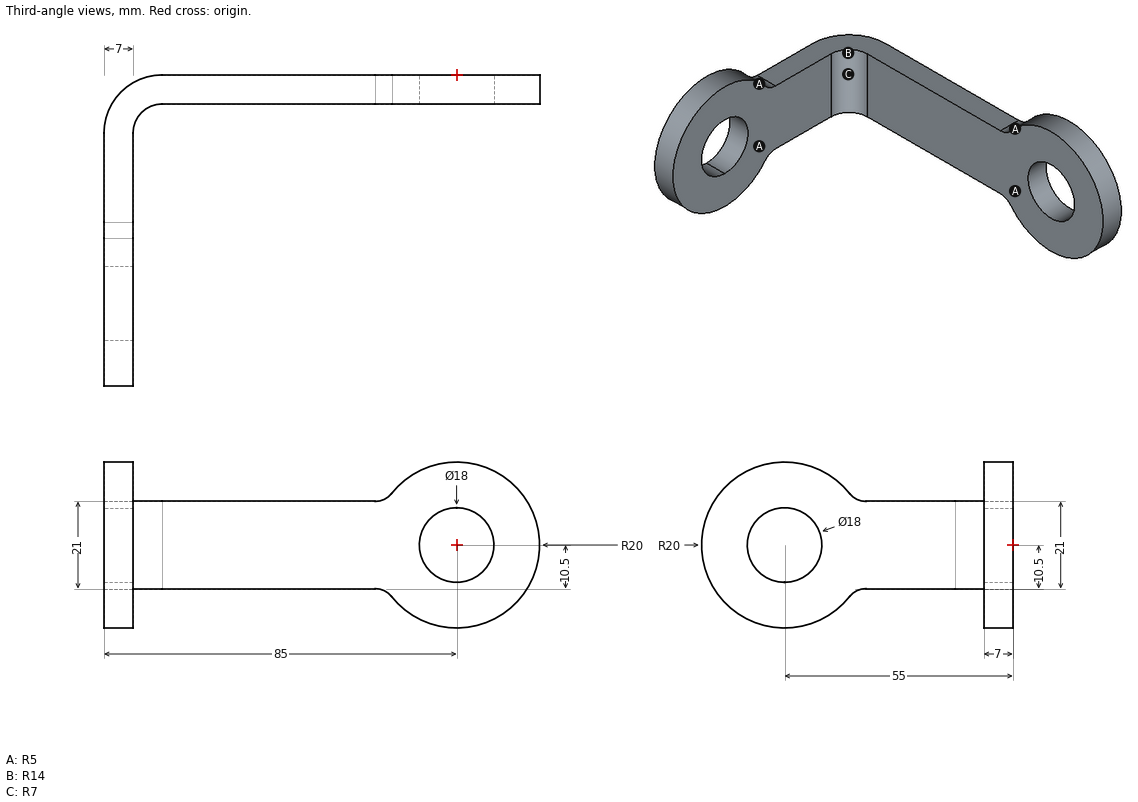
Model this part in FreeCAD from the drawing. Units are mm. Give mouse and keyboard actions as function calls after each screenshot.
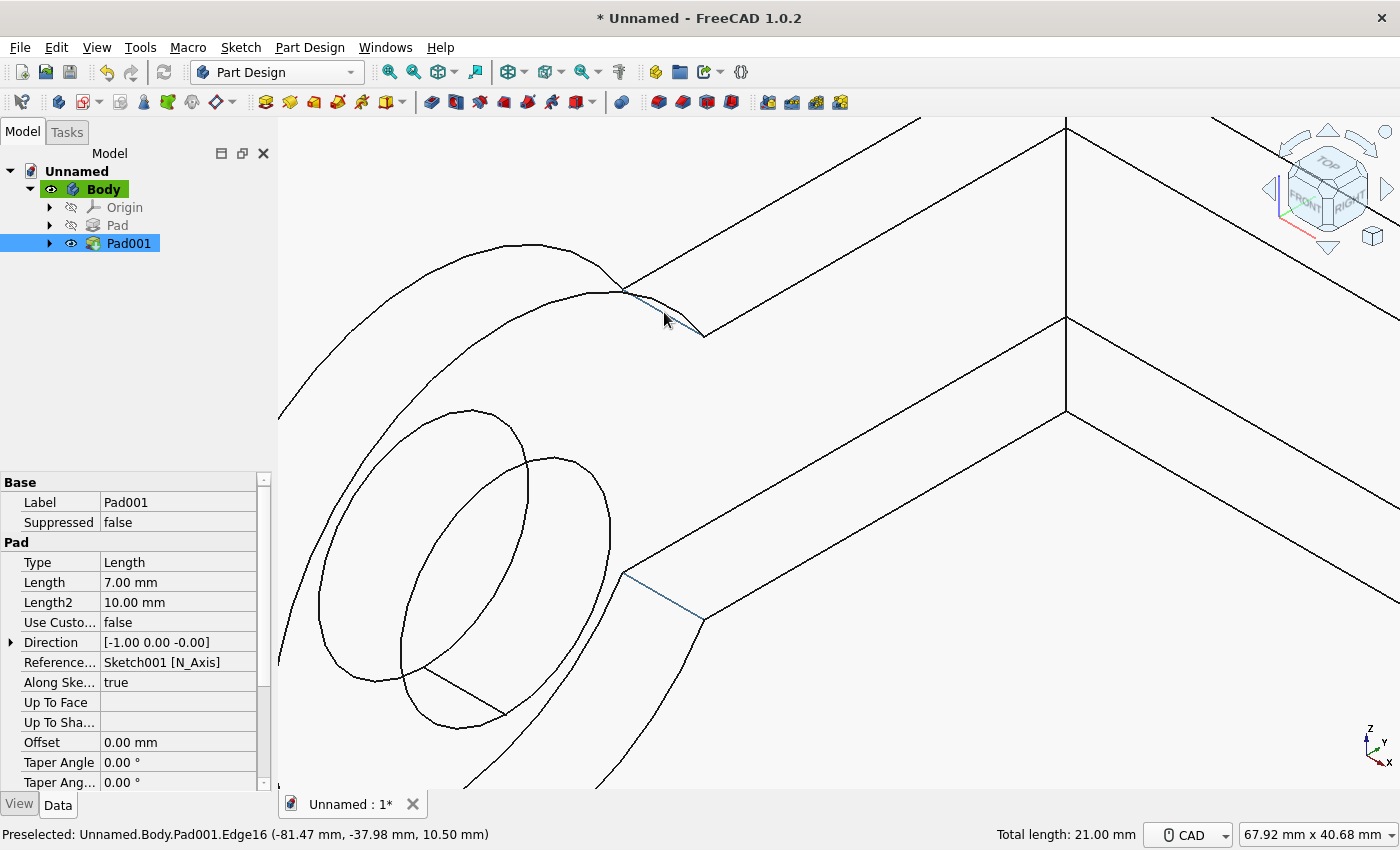
click(390, 72)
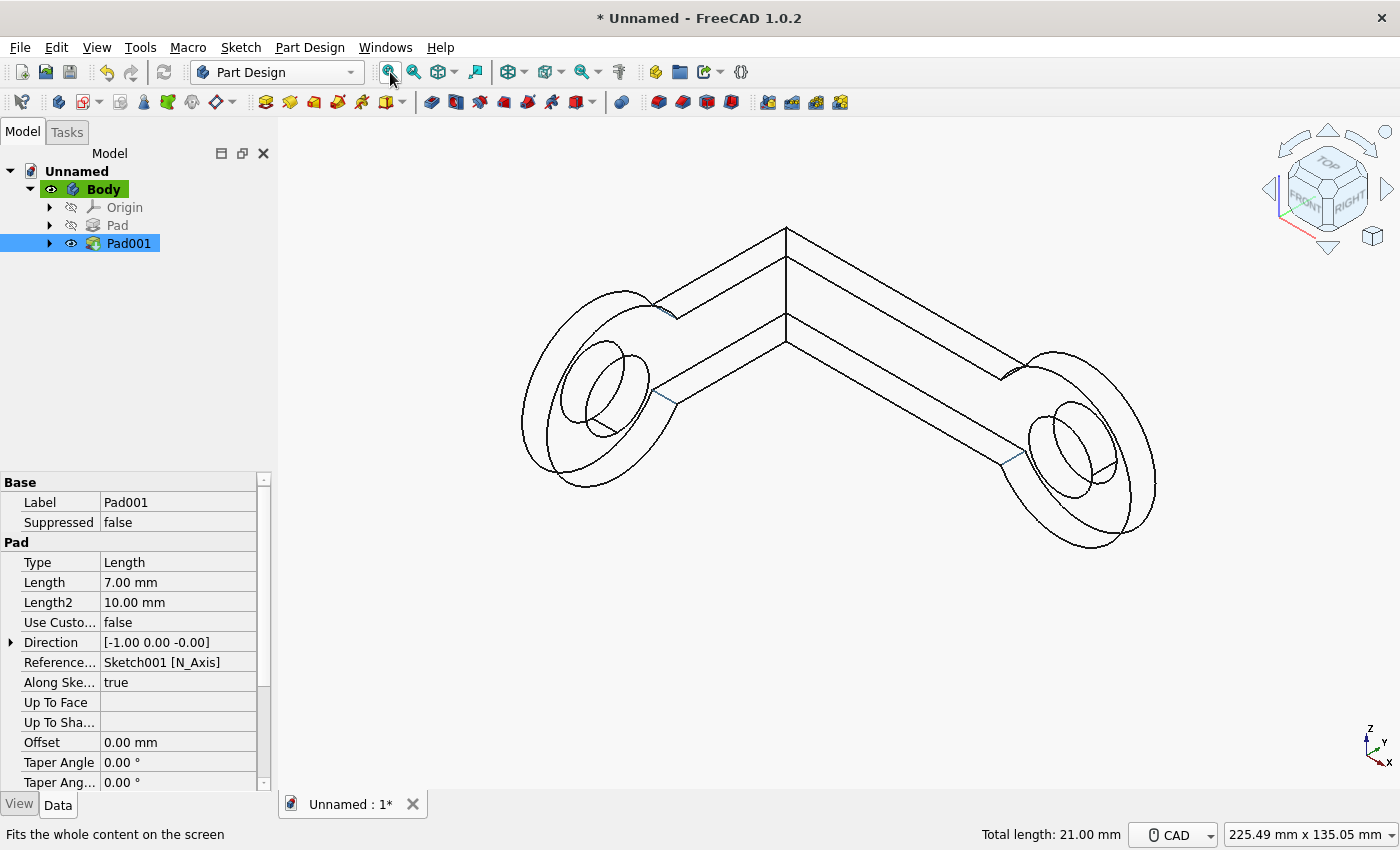
key(2)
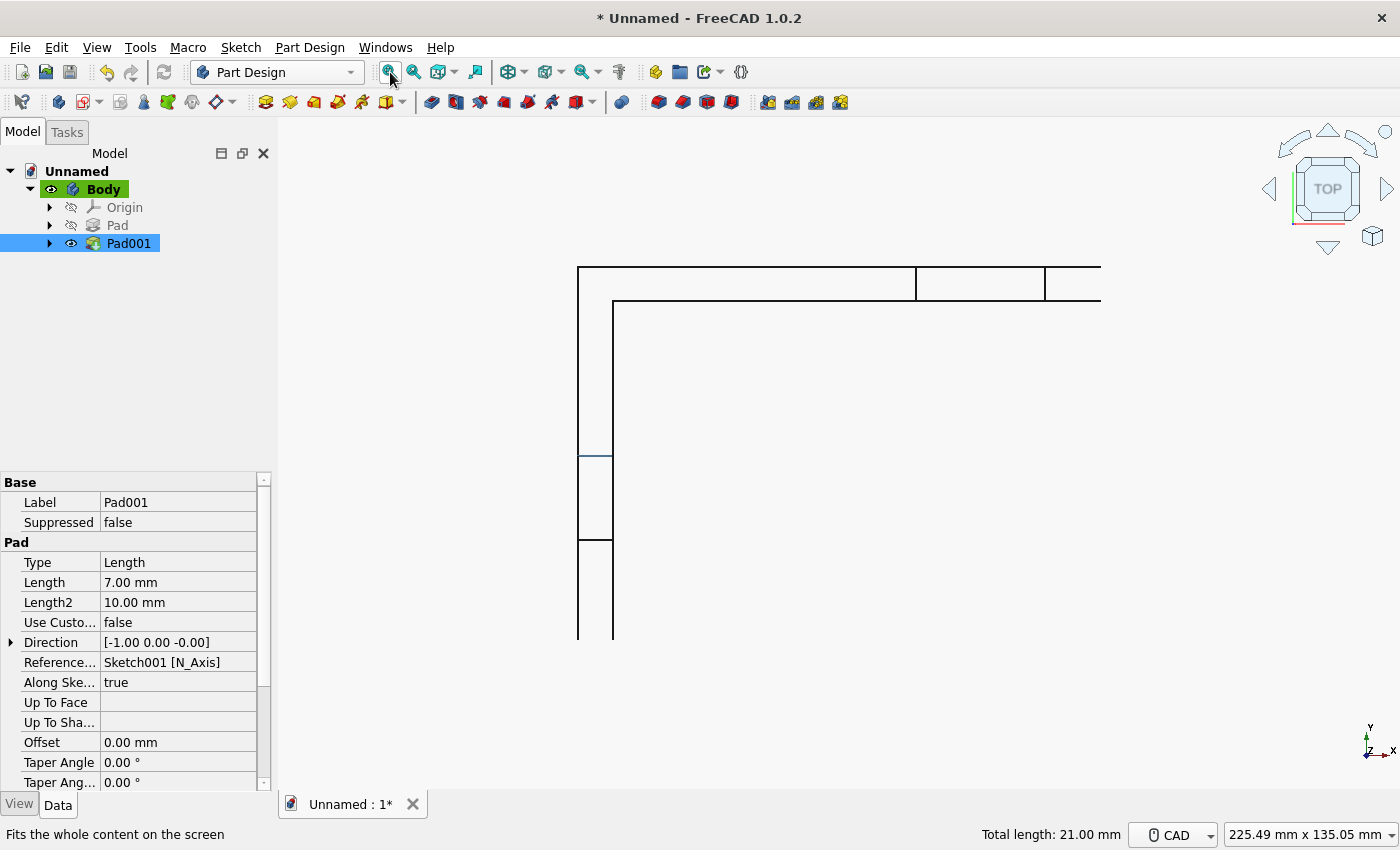
click(916, 283, ctrl)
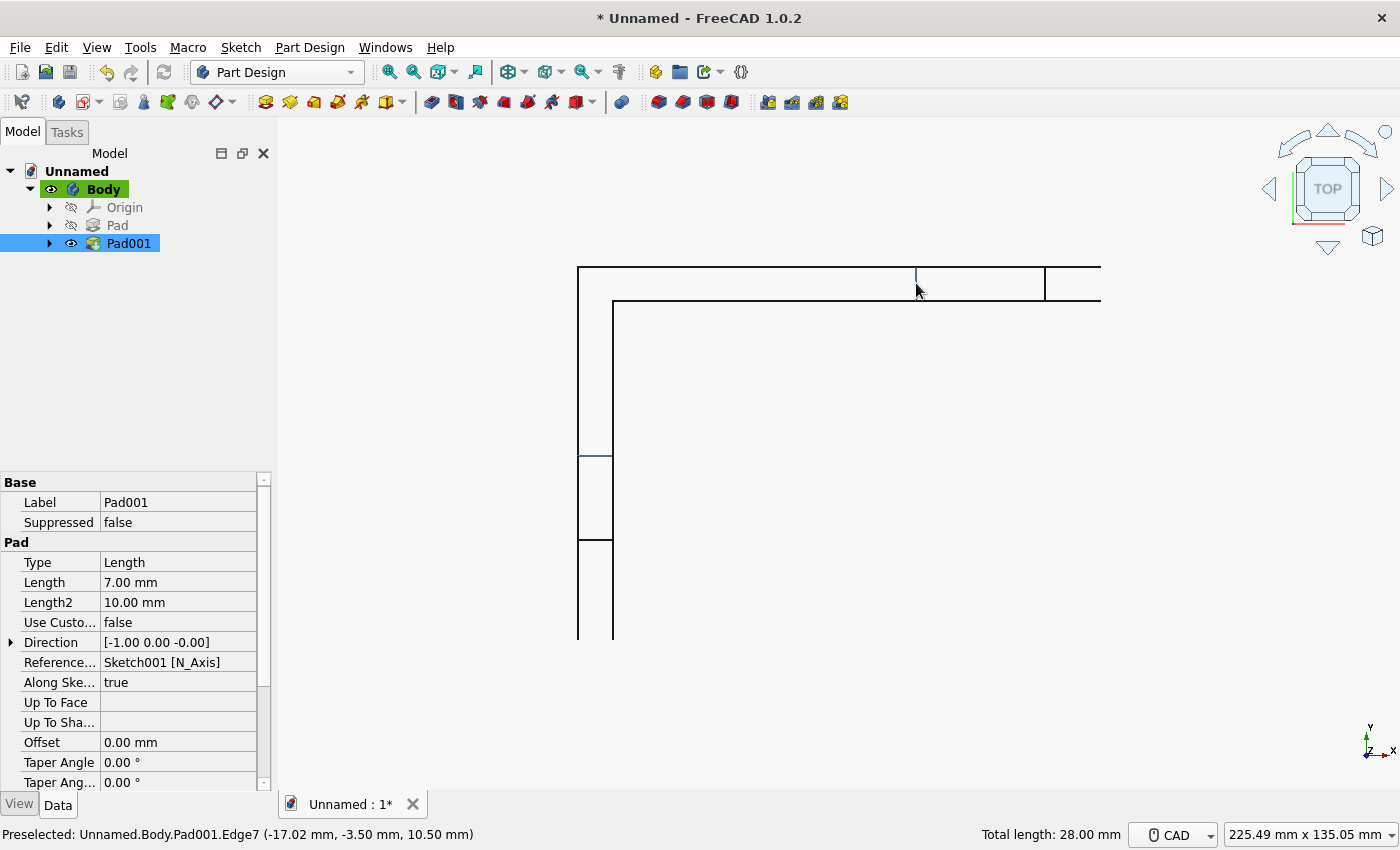
key(v)
key(1)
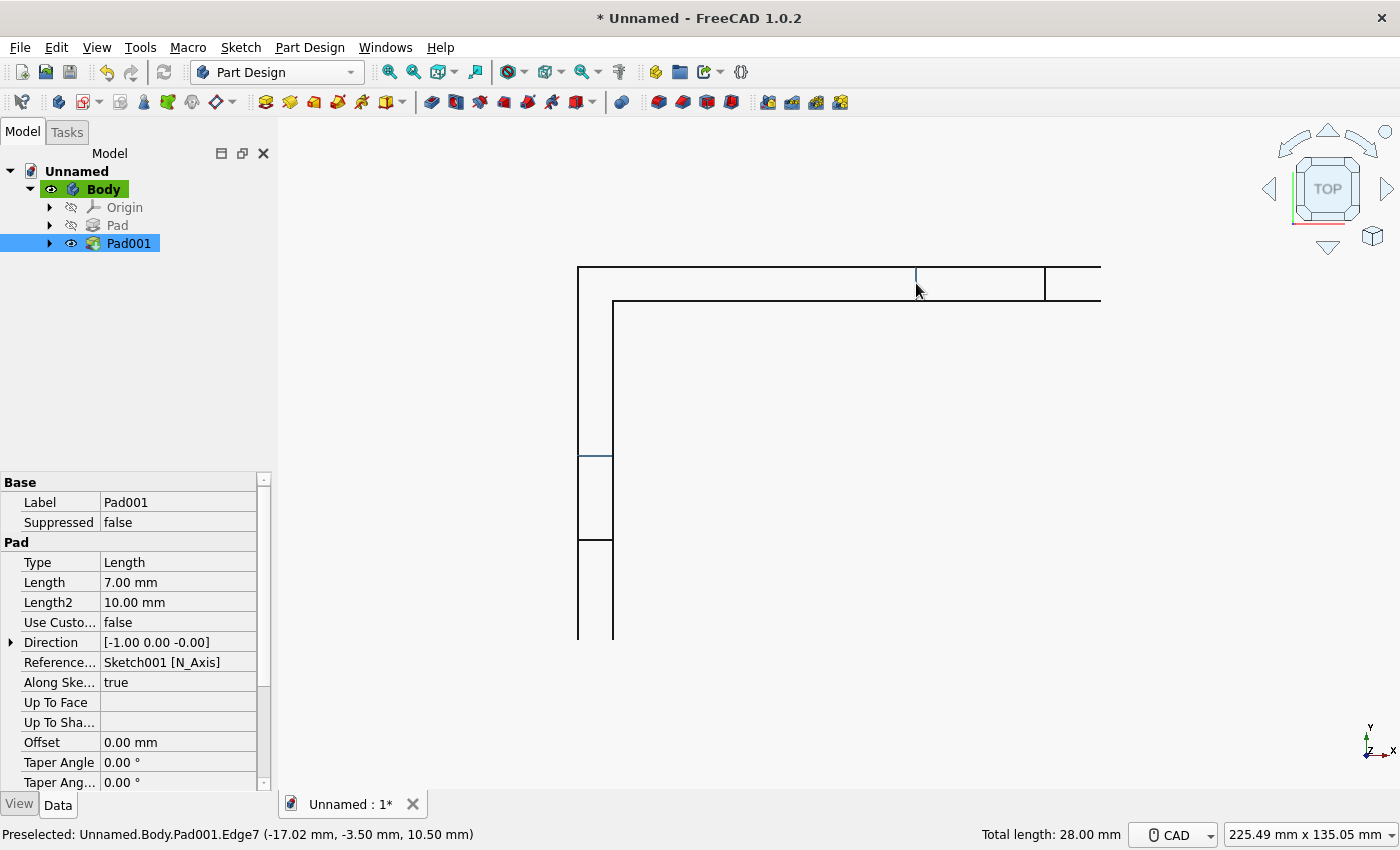
click(660, 102)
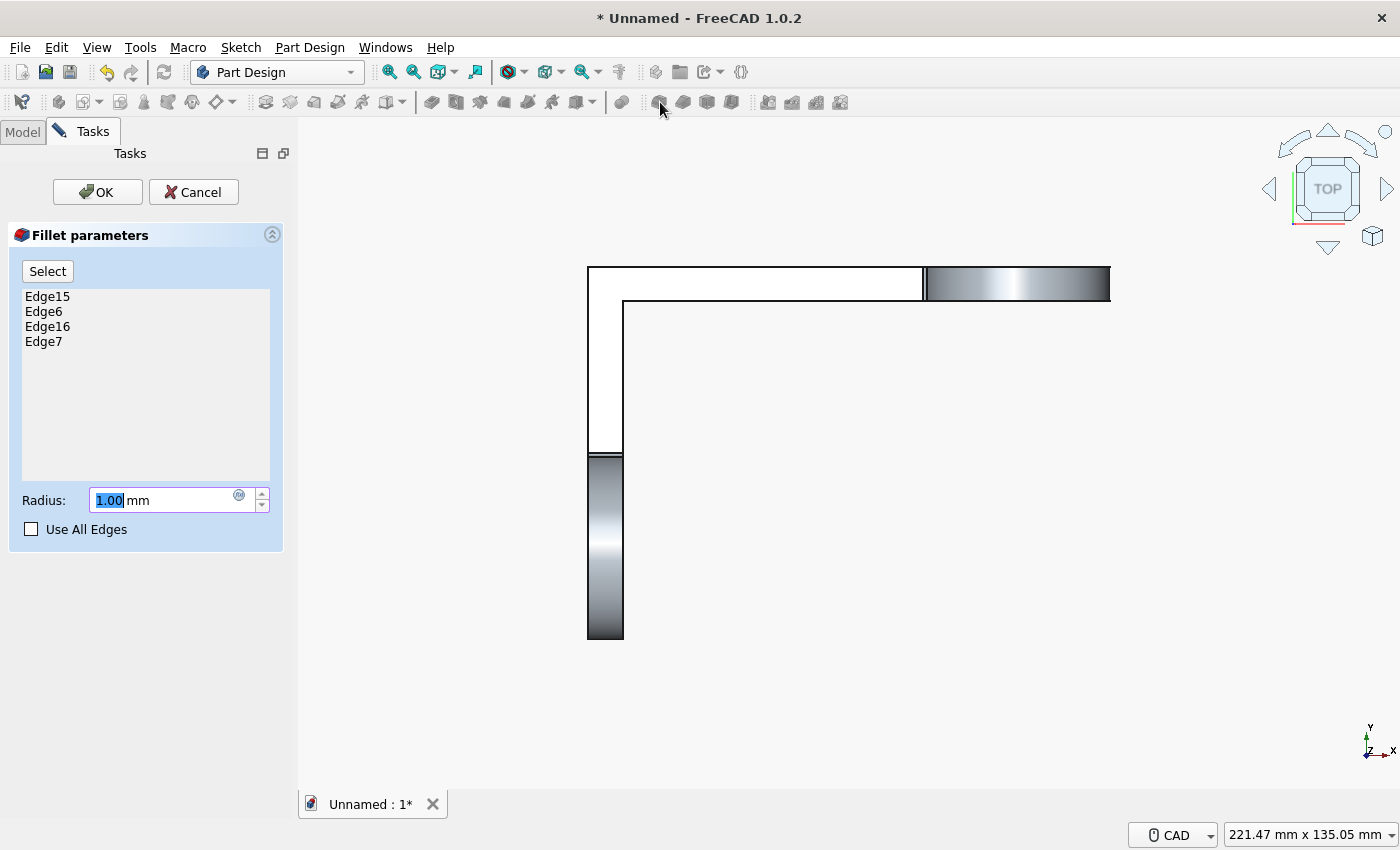
text(5)
key(Tab)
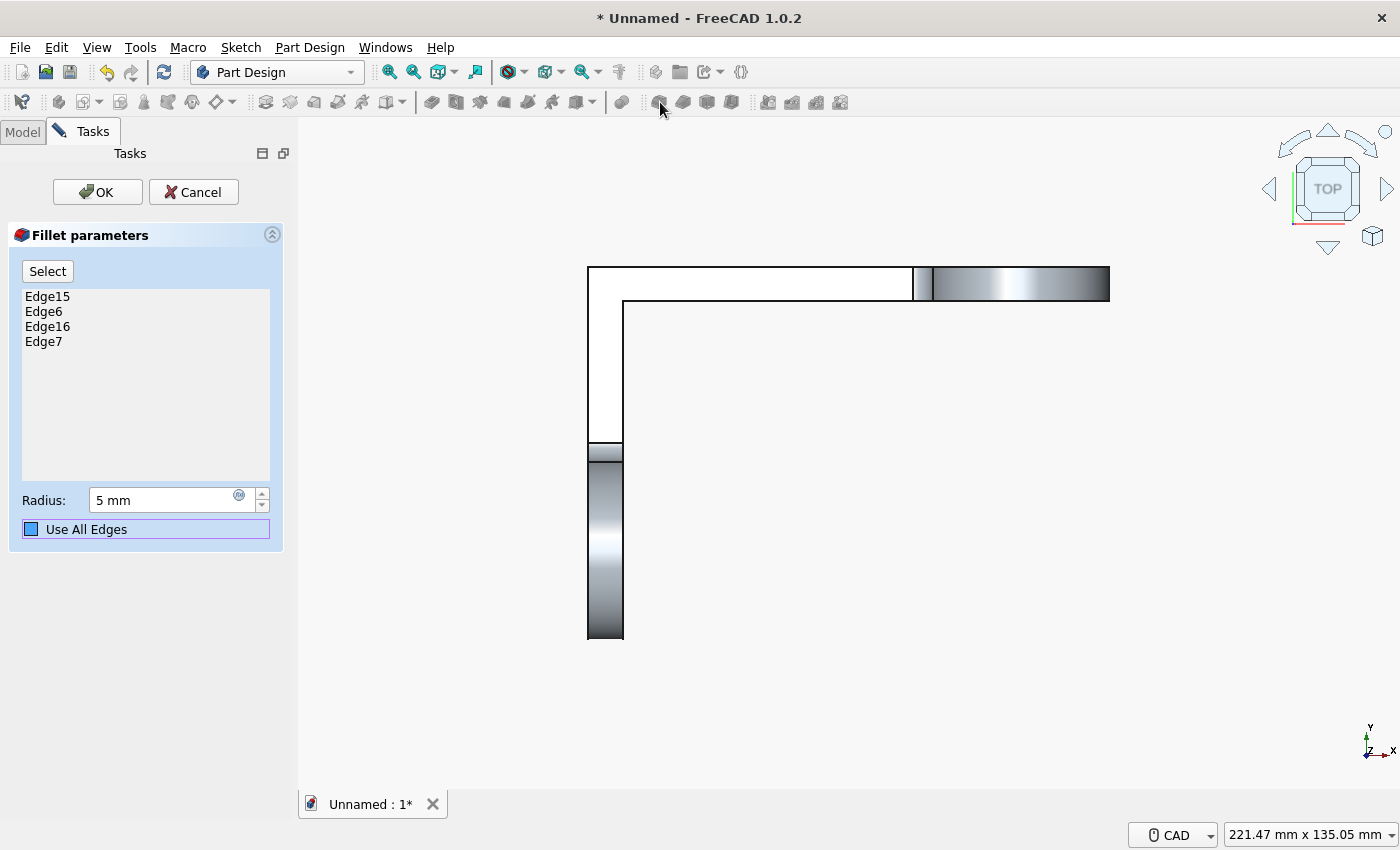
click(98, 192)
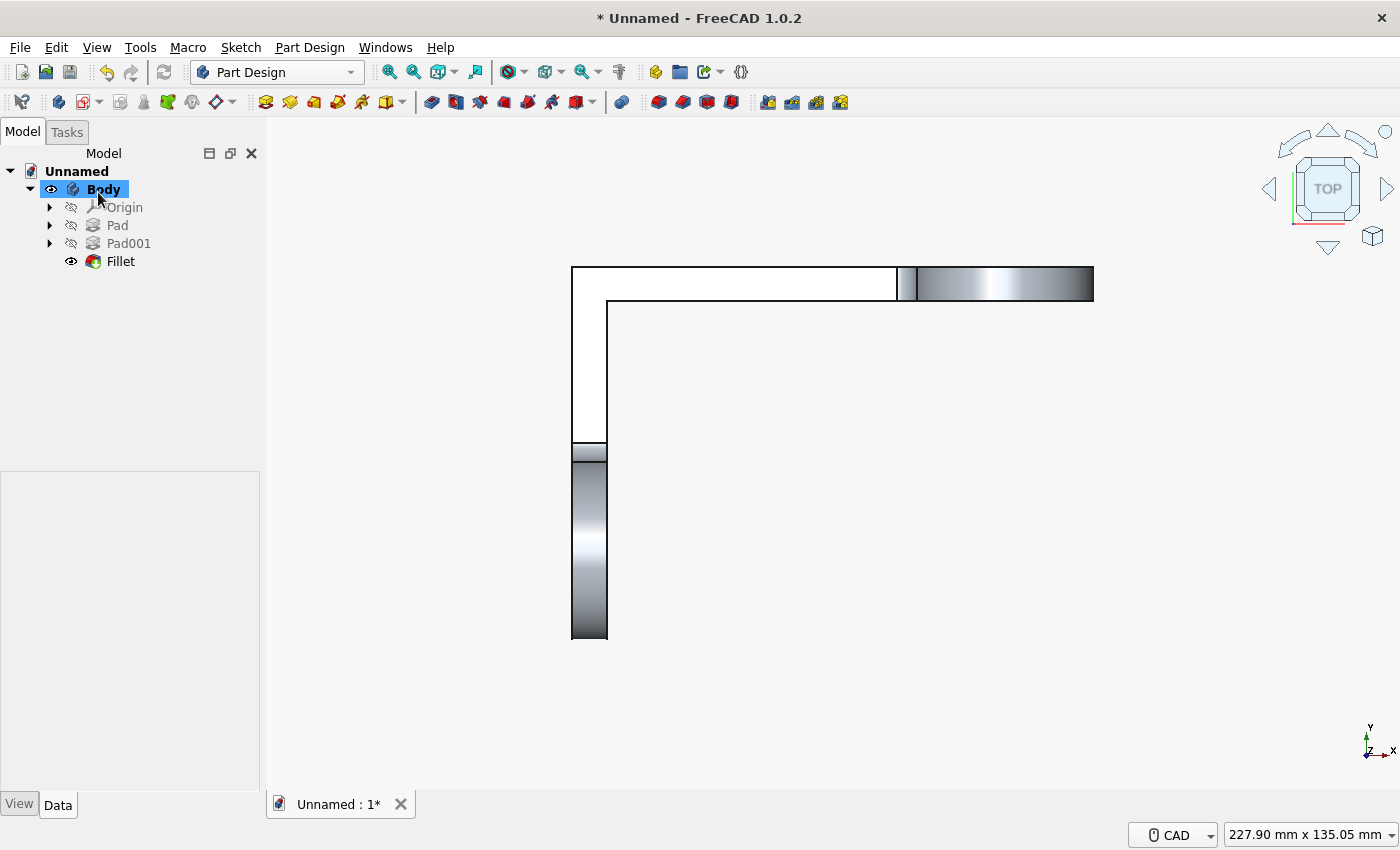
key(0)